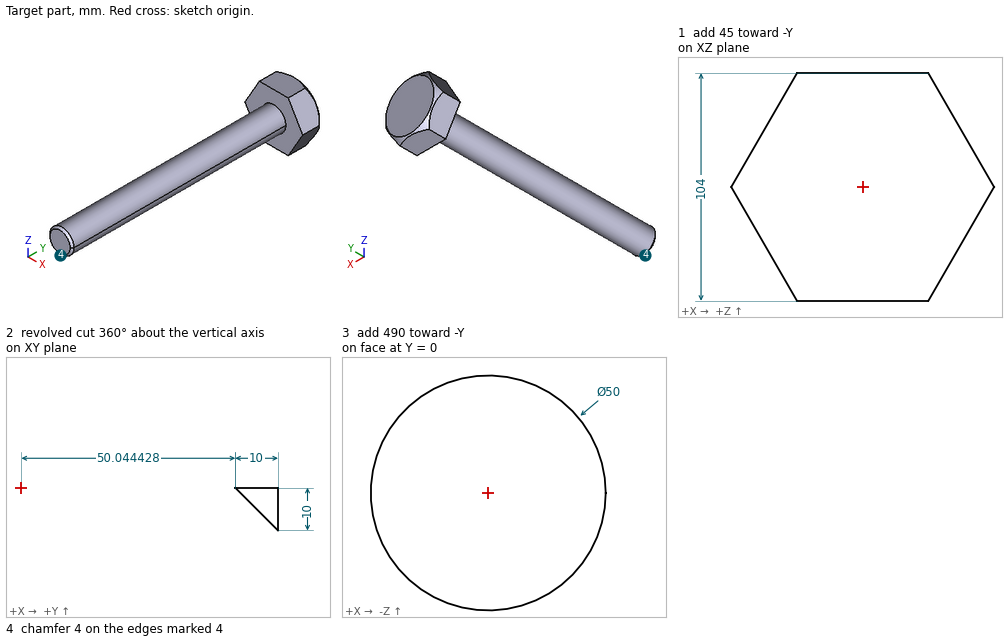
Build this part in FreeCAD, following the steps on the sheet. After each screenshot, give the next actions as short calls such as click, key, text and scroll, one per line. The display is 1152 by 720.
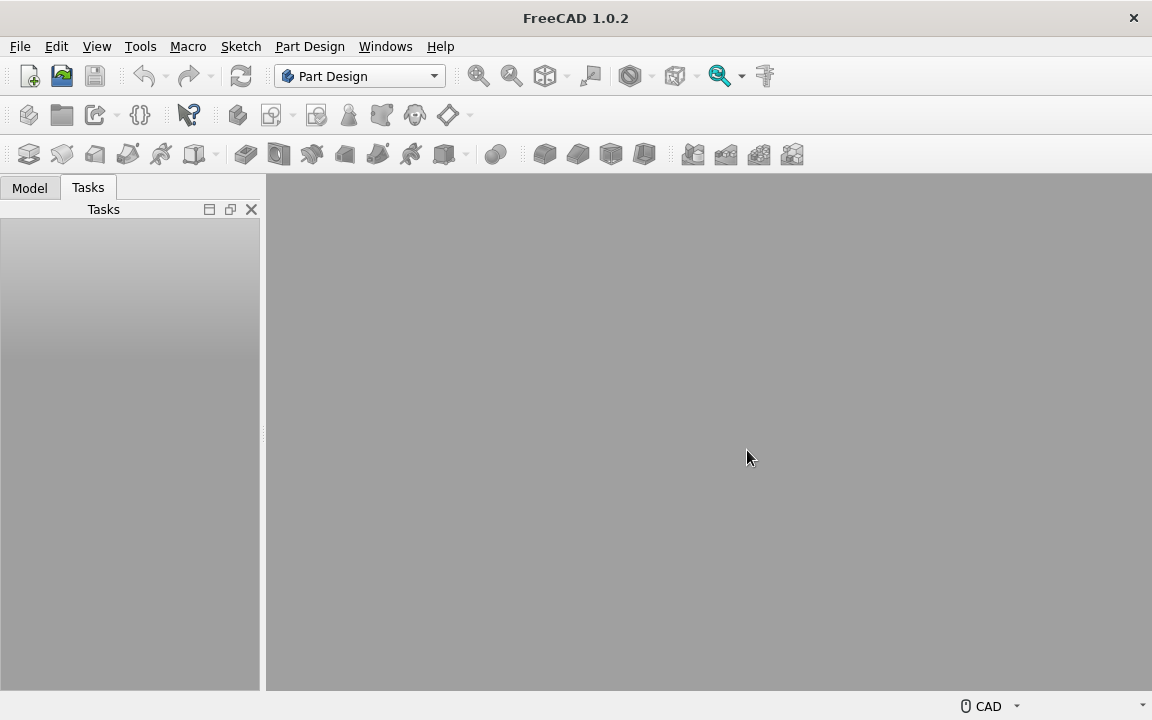
click(29, 76)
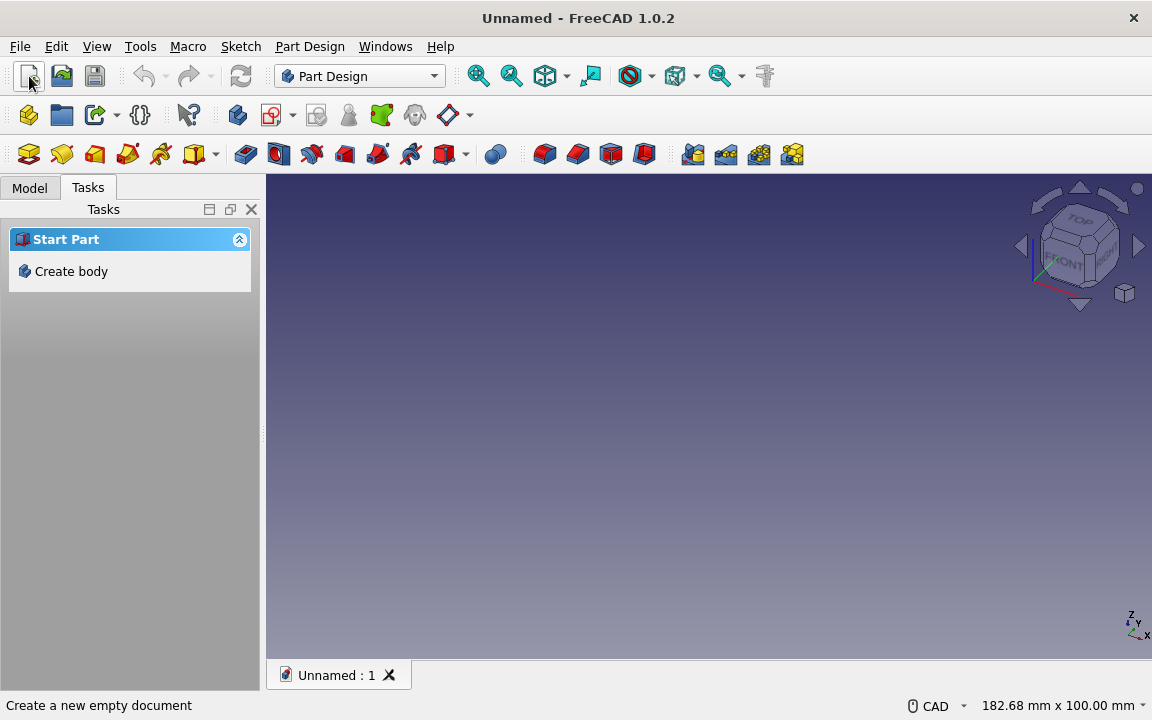
click(270, 116)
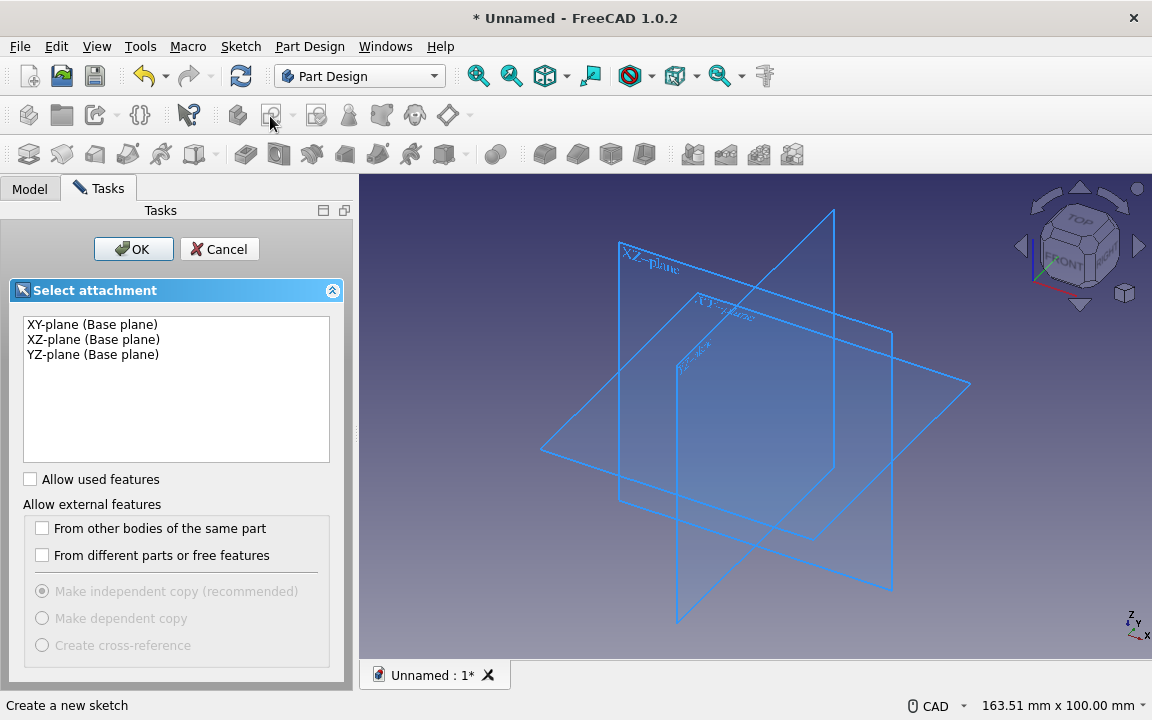
click(84, 340)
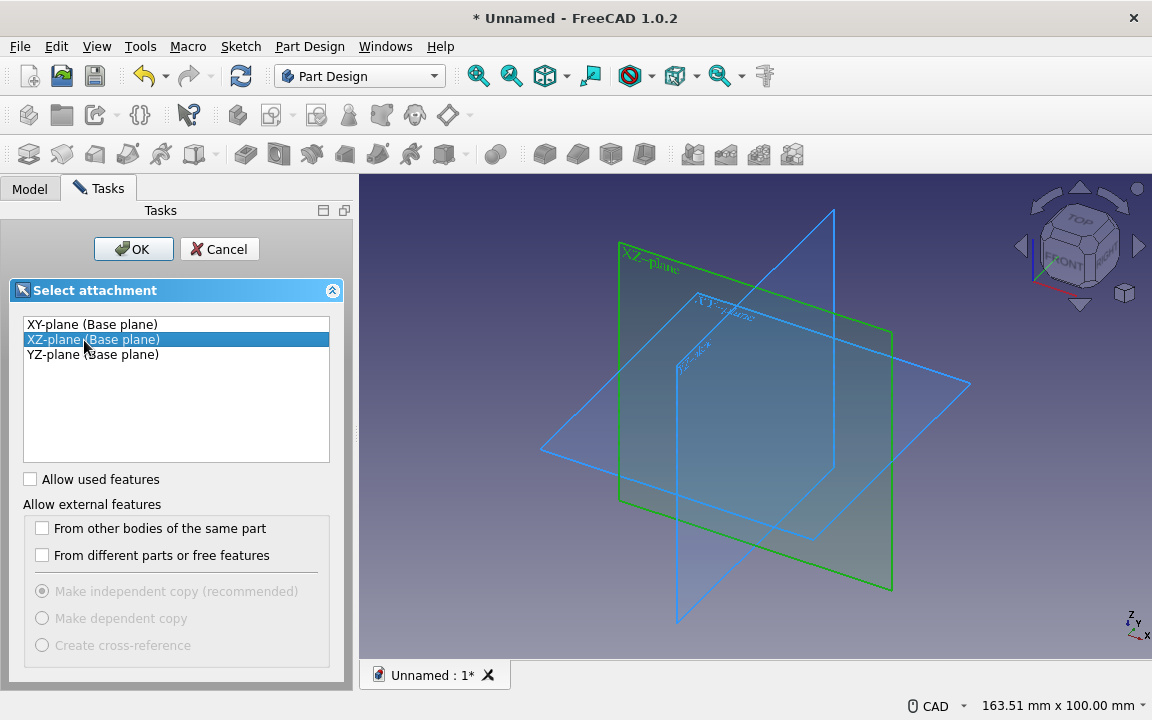
click(134, 249)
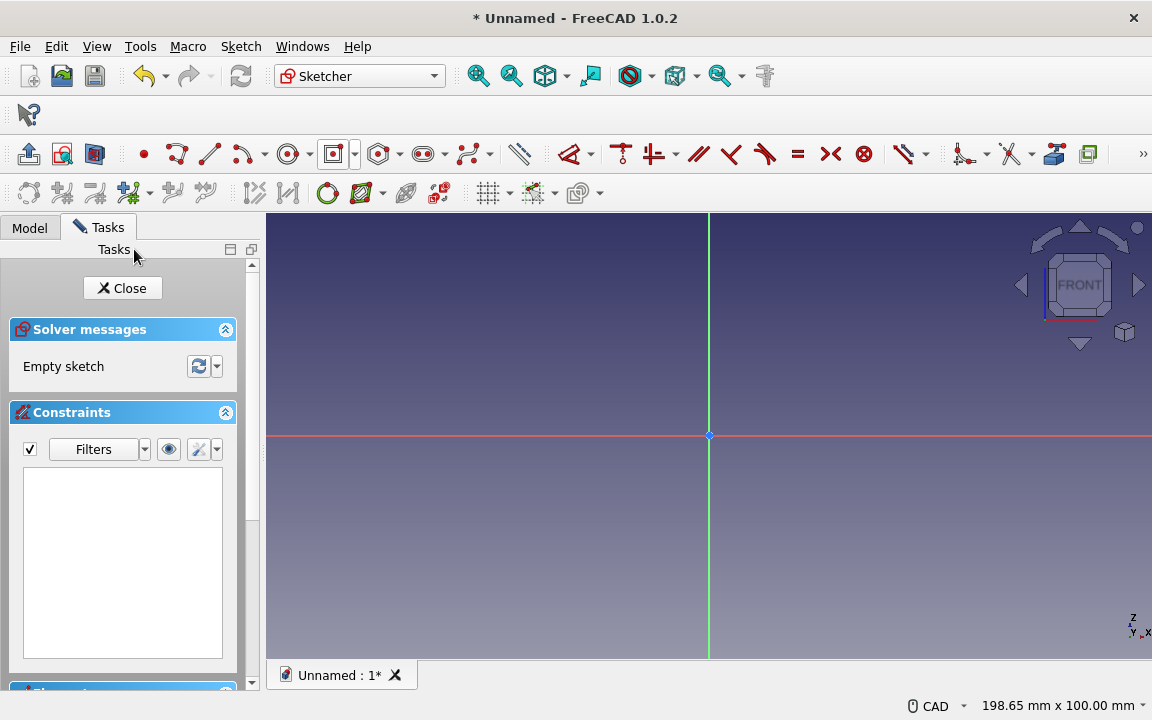
scroll(557, 436, down, 3)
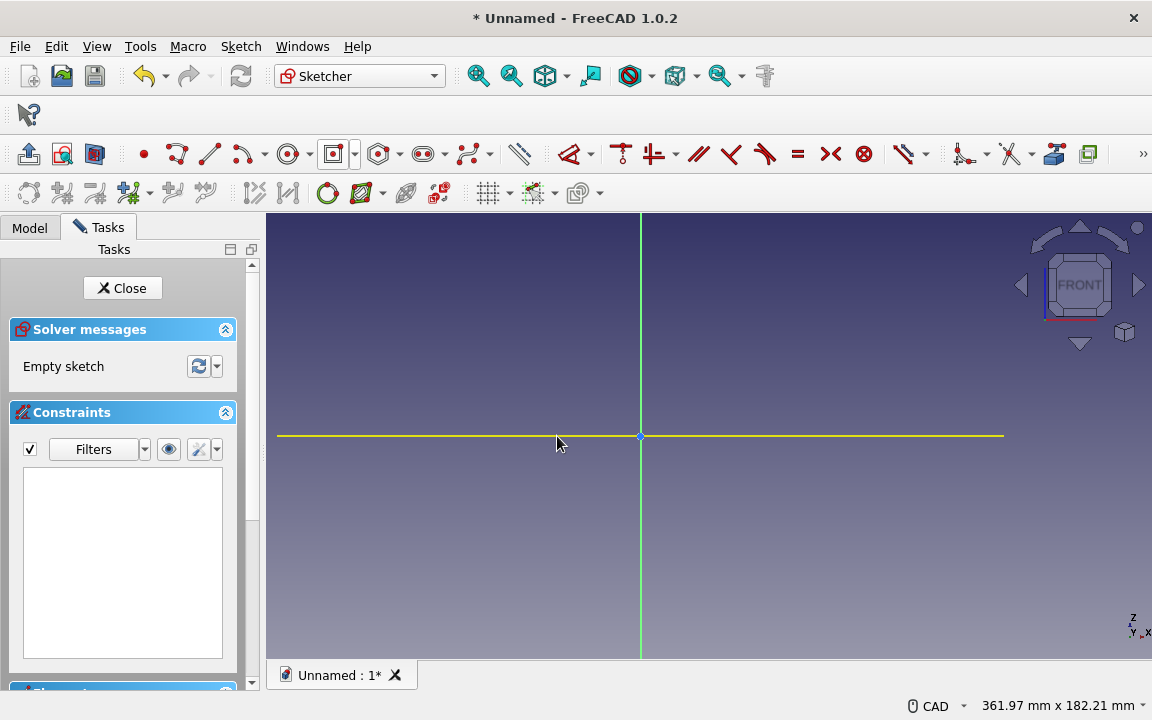
click(378, 154)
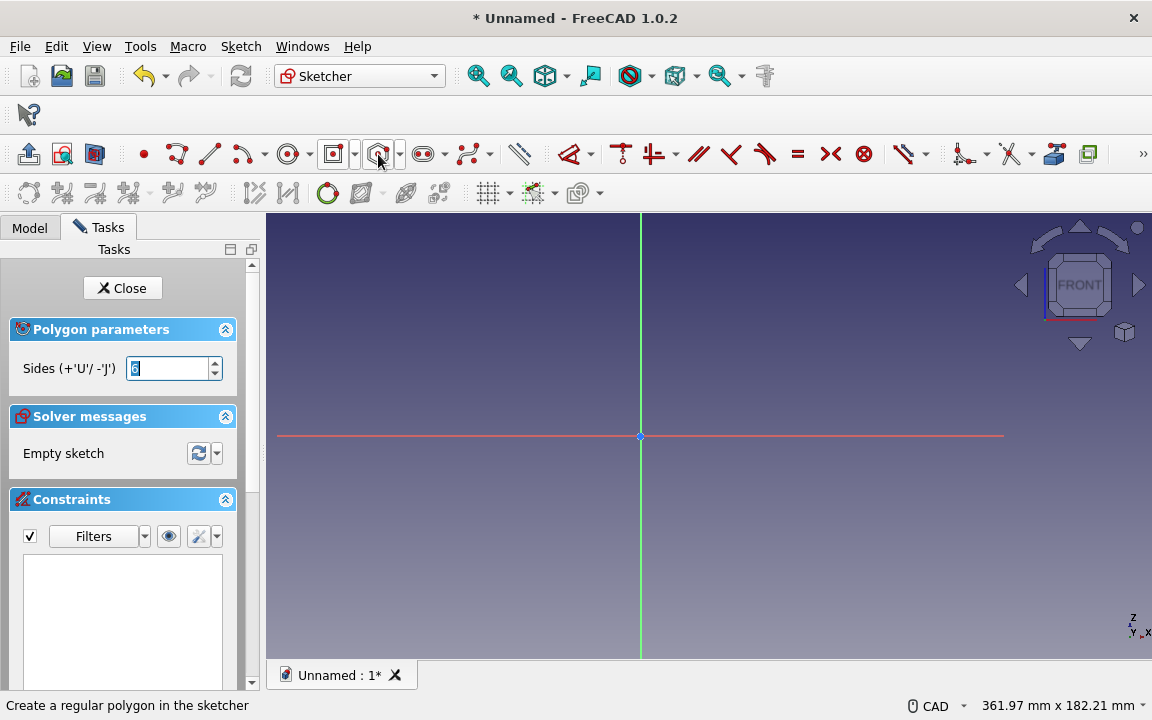
click(641, 436)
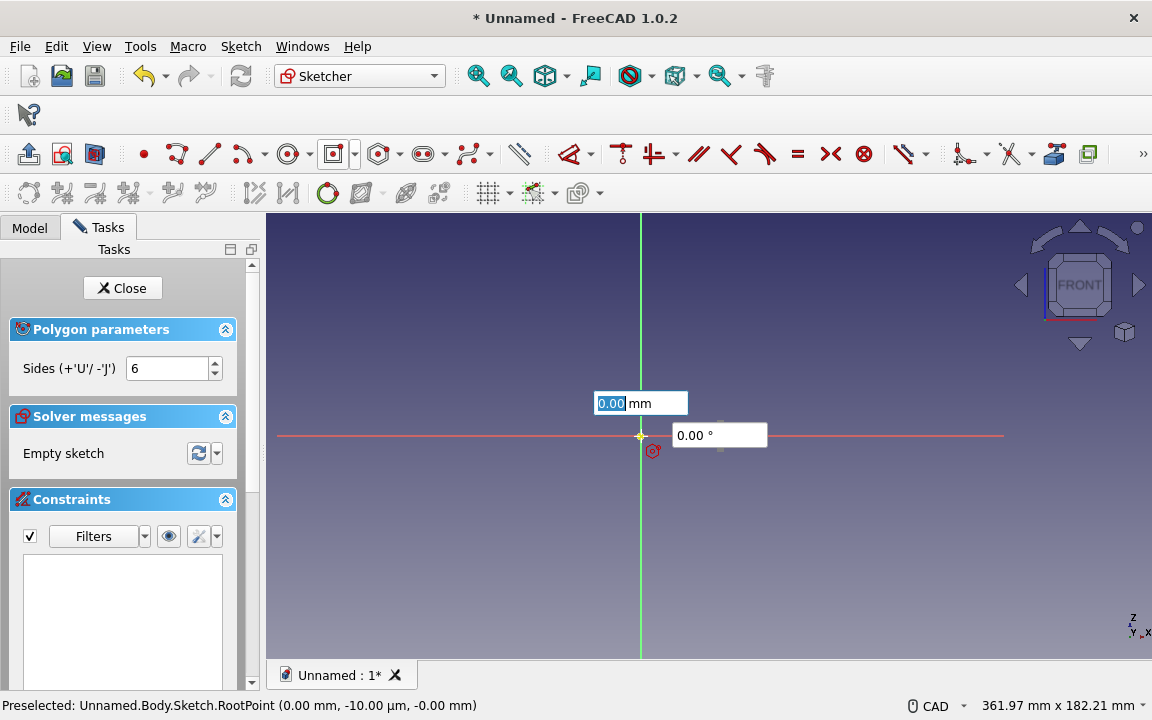
click(788, 436)
right_click(788, 436)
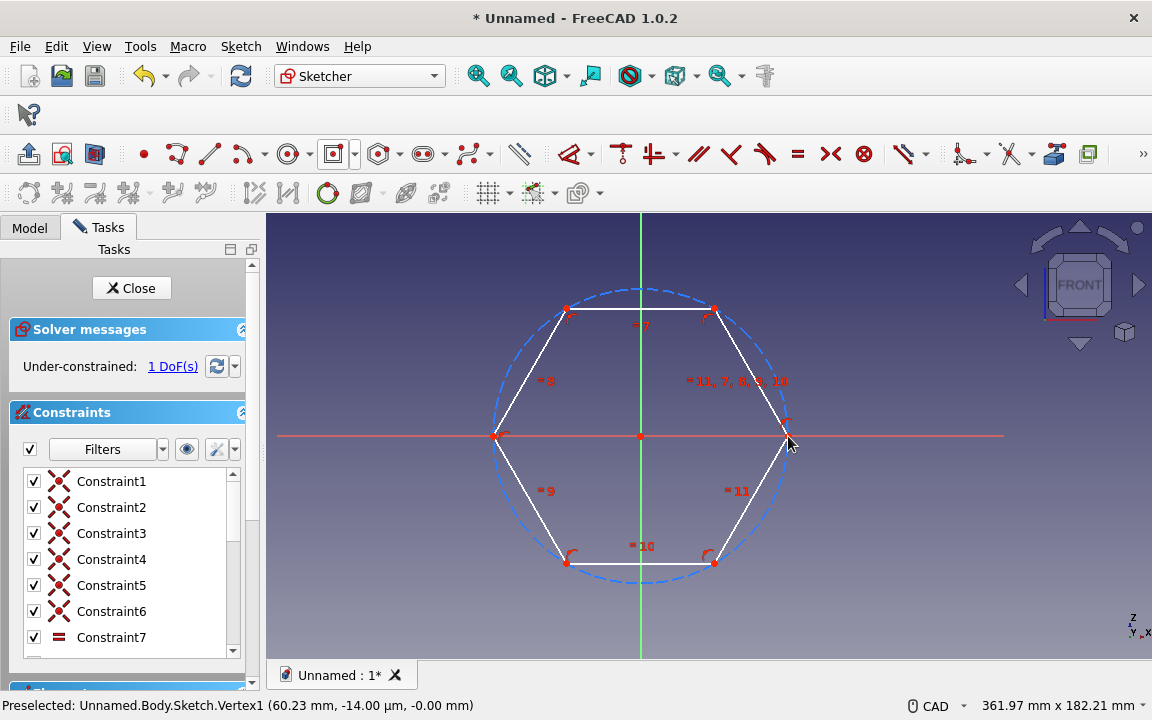
click(567, 564)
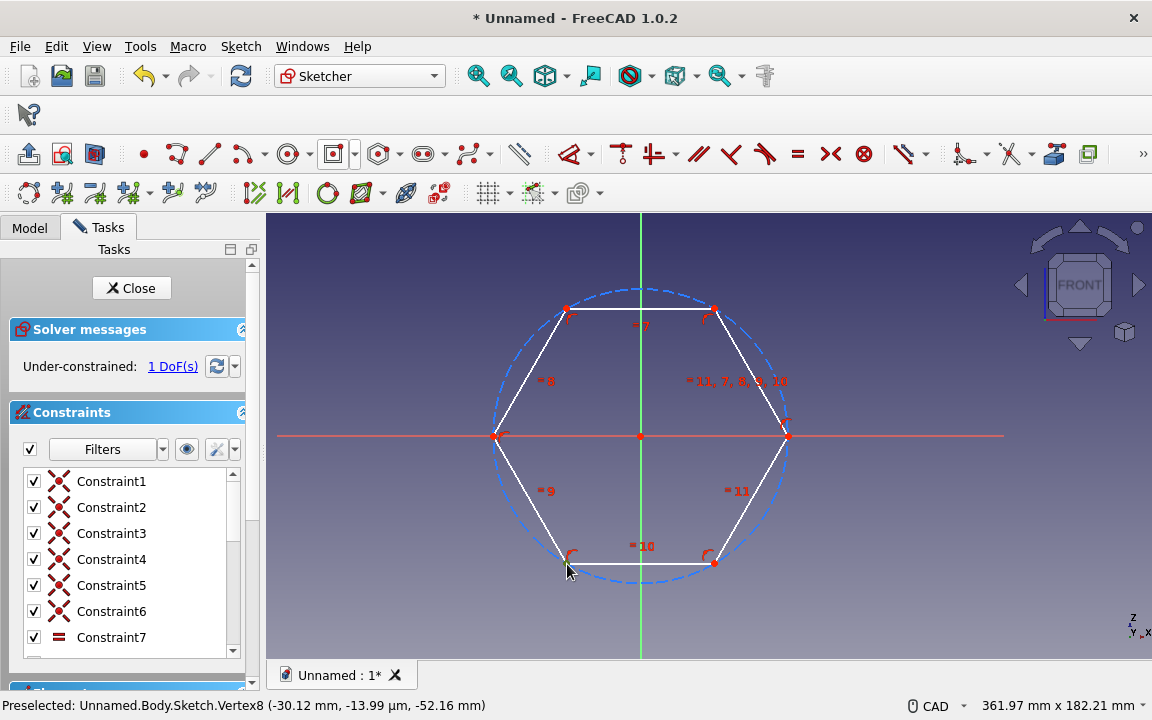
click(714, 309)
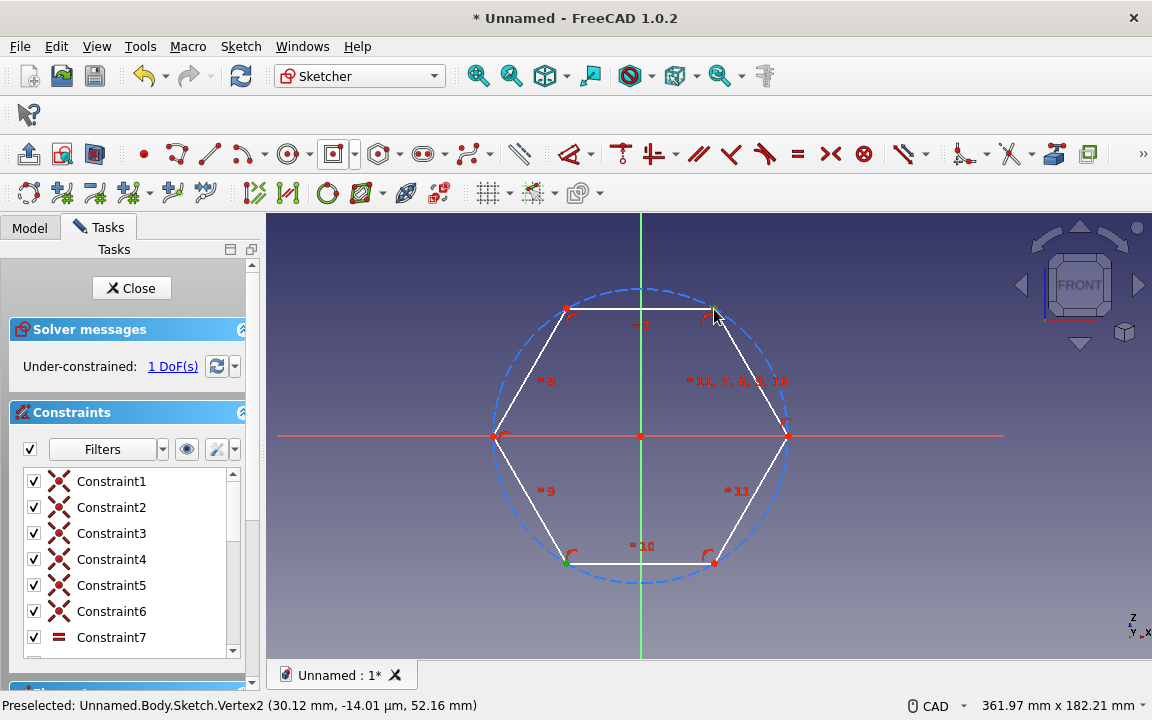
key(i)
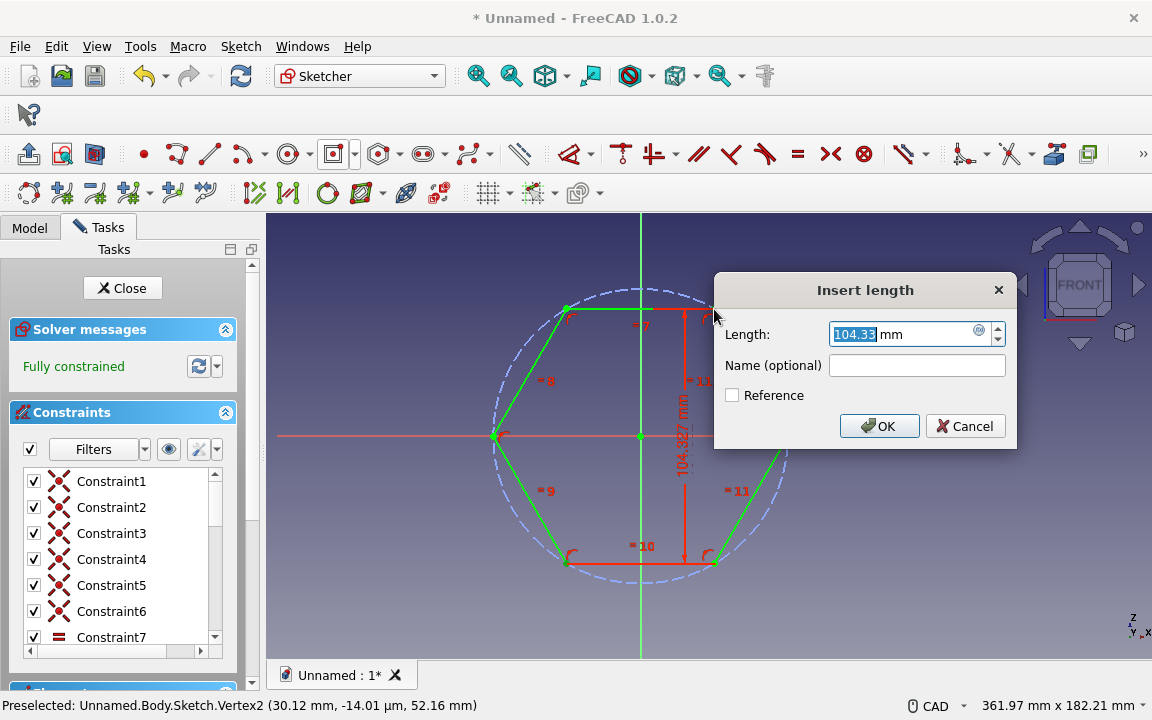
text(104)
key(Return)